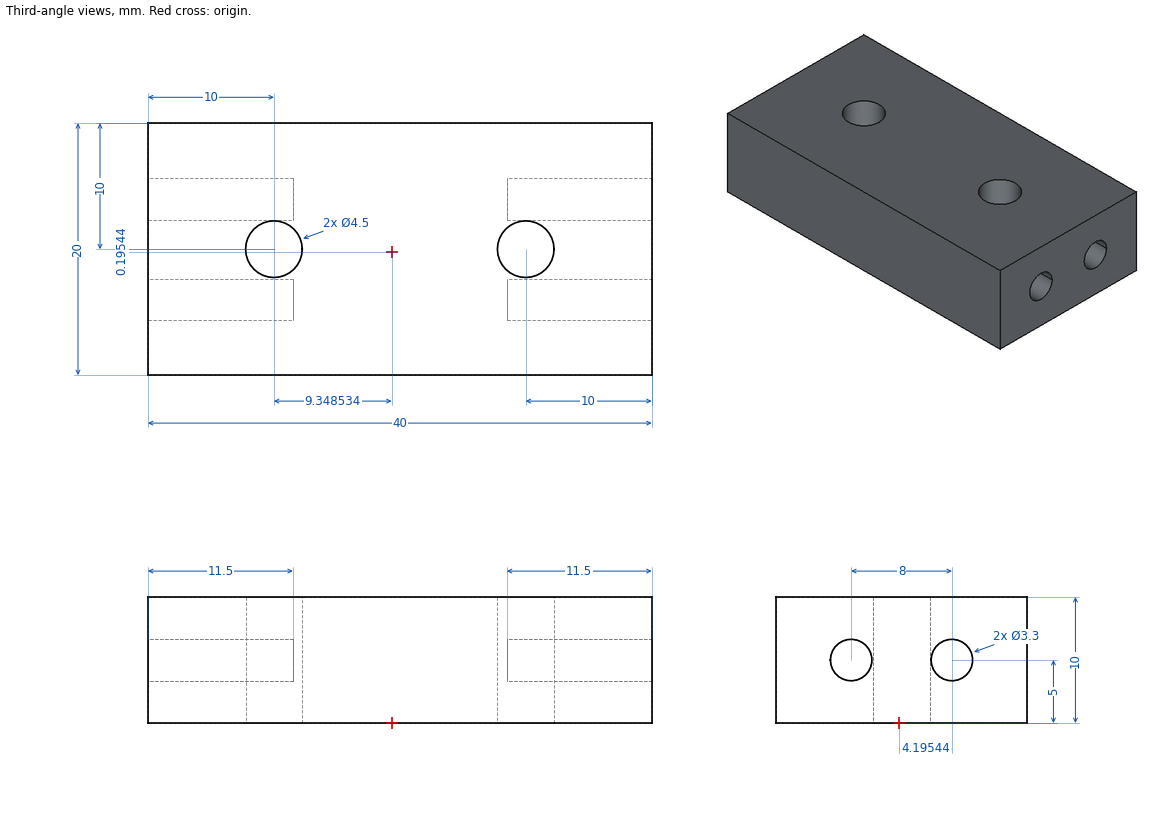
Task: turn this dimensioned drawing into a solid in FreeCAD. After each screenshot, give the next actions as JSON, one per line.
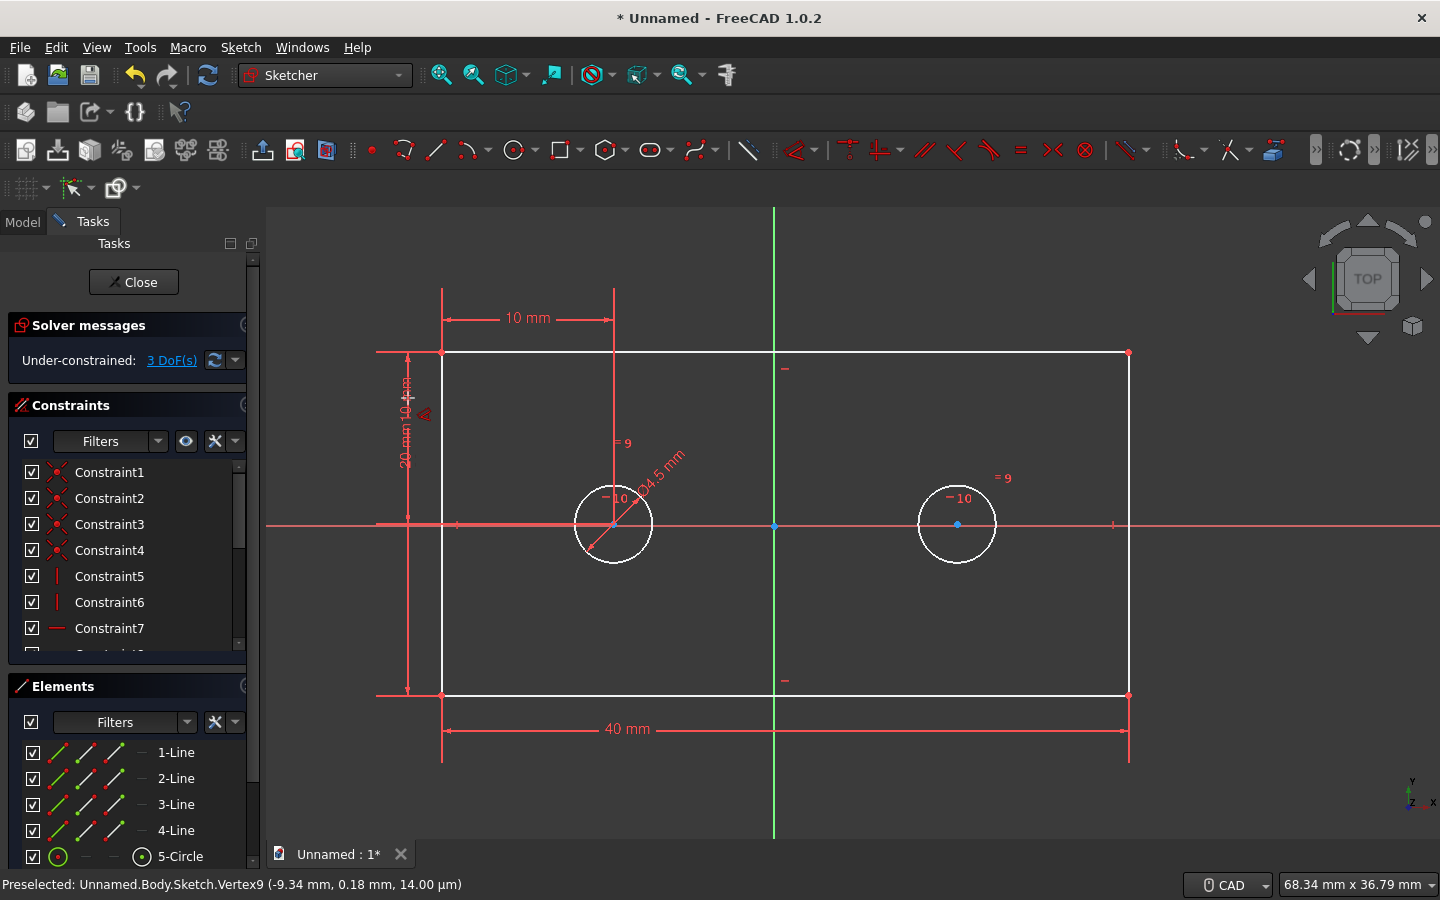
{"action": "left_click", "coordinate": [1129, 696]}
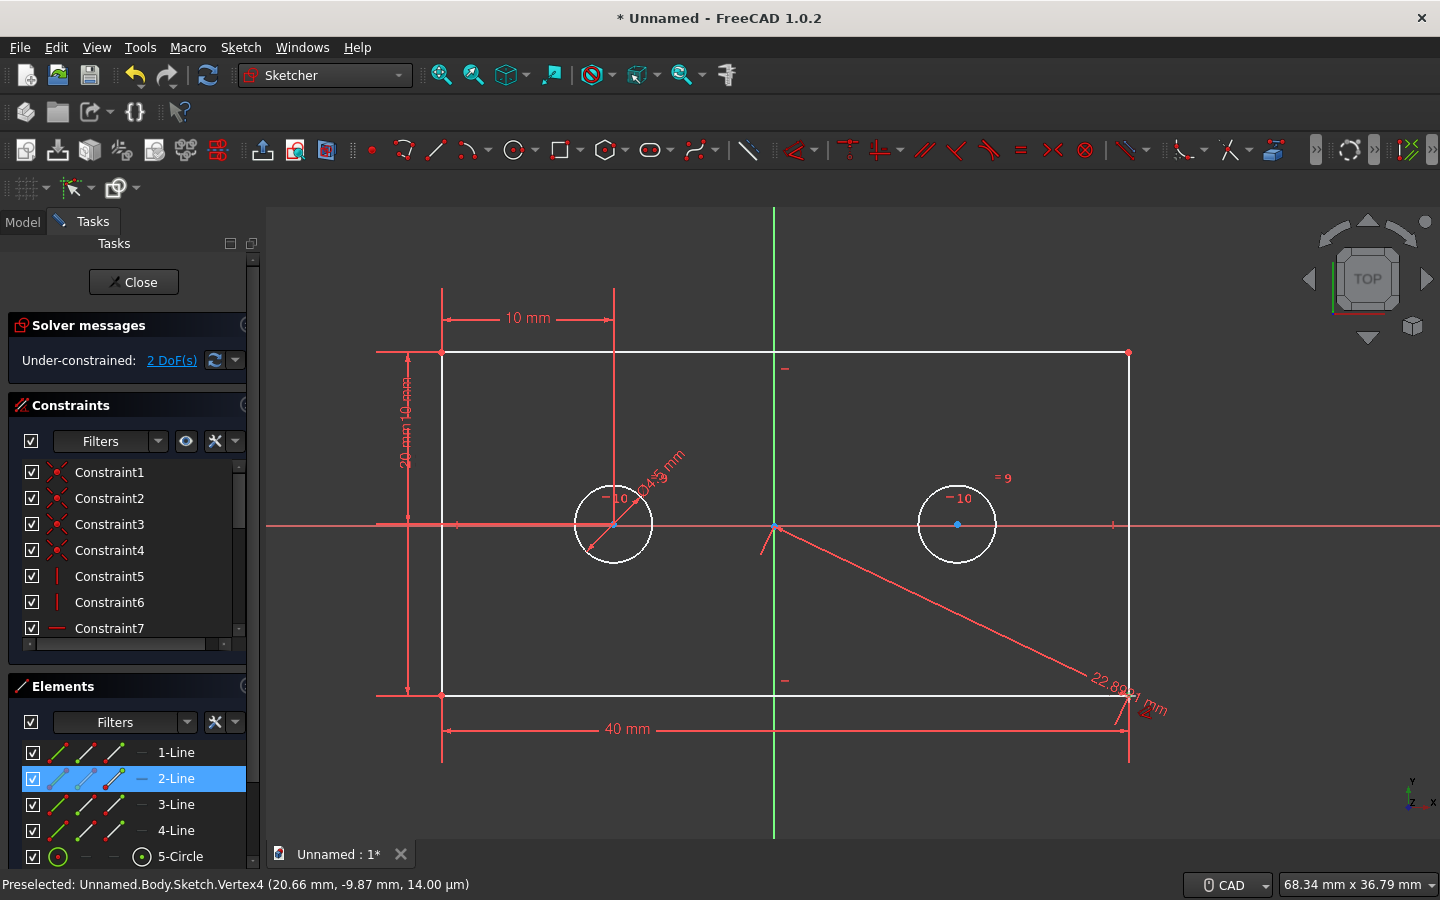
{"action": "left_click", "coordinate": [957, 524]}
{"action": "left_click", "coordinate": [1043, 730]}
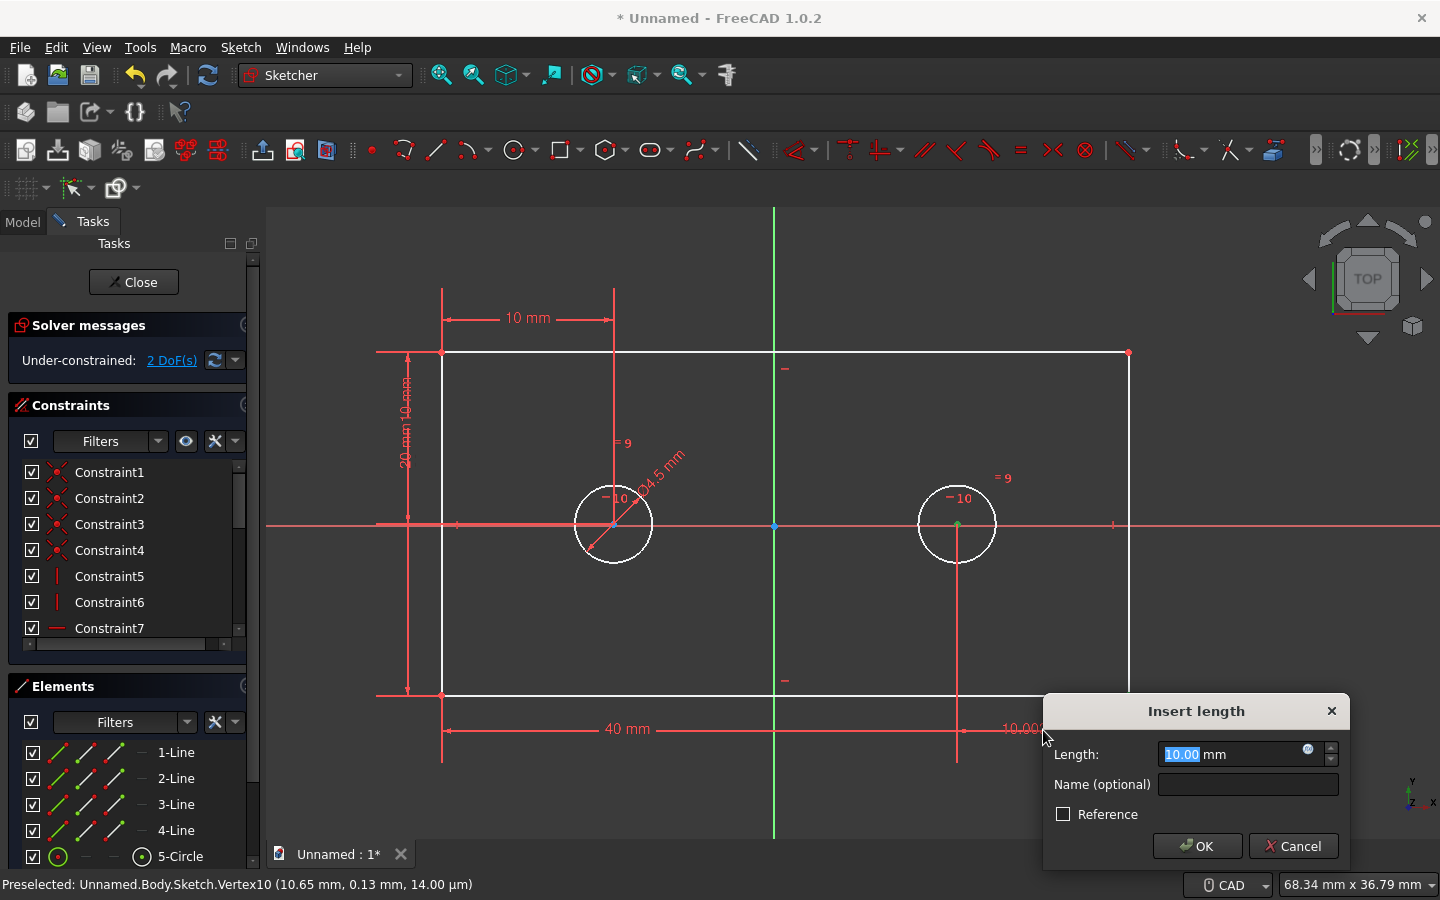
{"action": "type", "text": "10"}
{"action": "key", "text": "Return"}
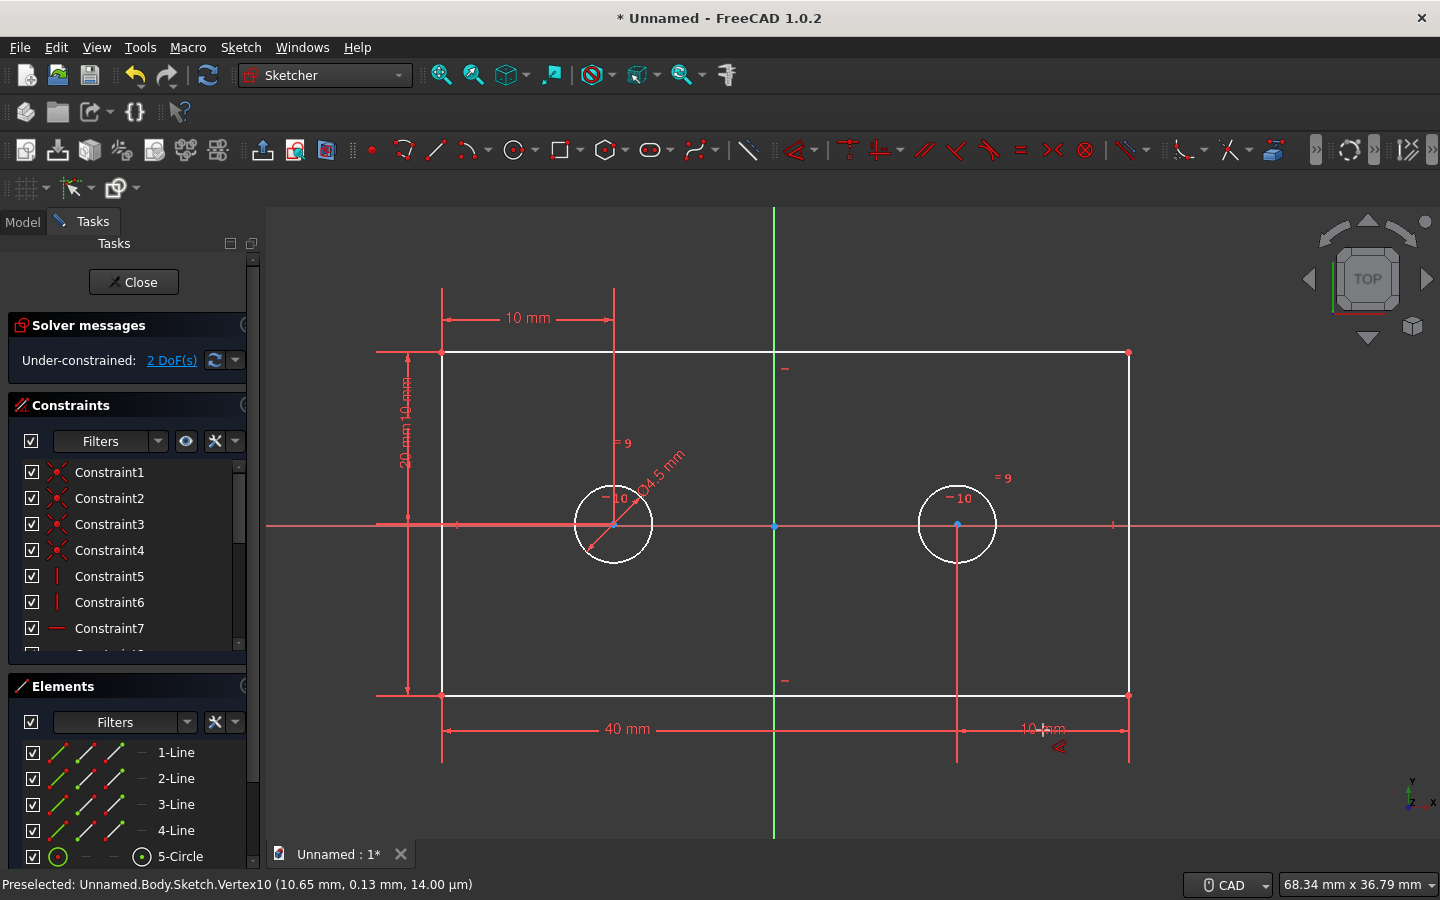
{"action": "scroll", "coordinate": [614, 524], "scroll_direction": "up", "scroll_amount": 13}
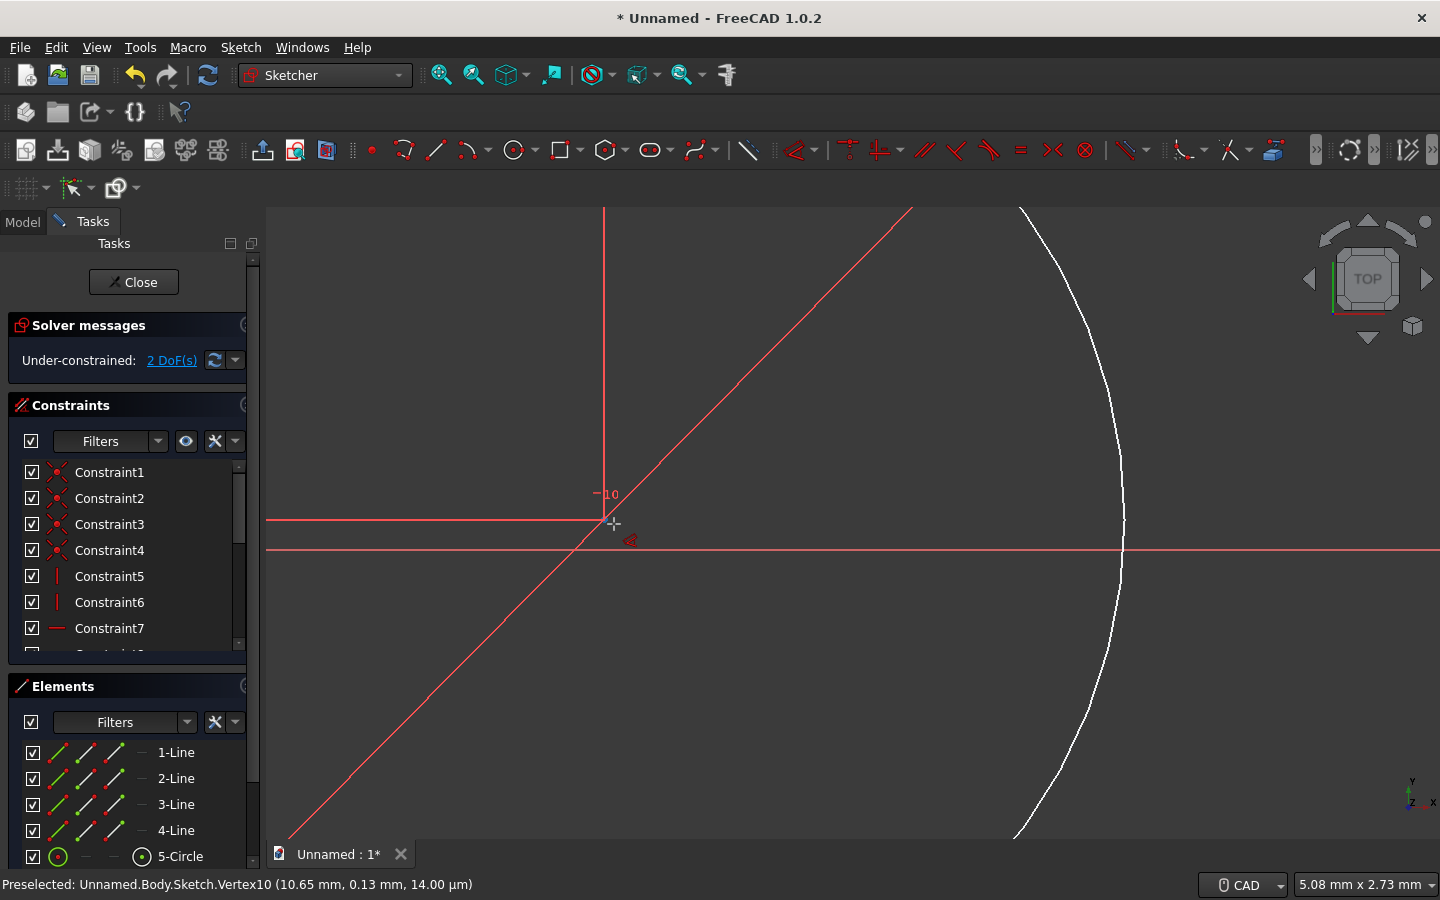
{"action": "left_click", "coordinate": [604, 520]}
{"action": "left_click", "coordinate": [570, 535]}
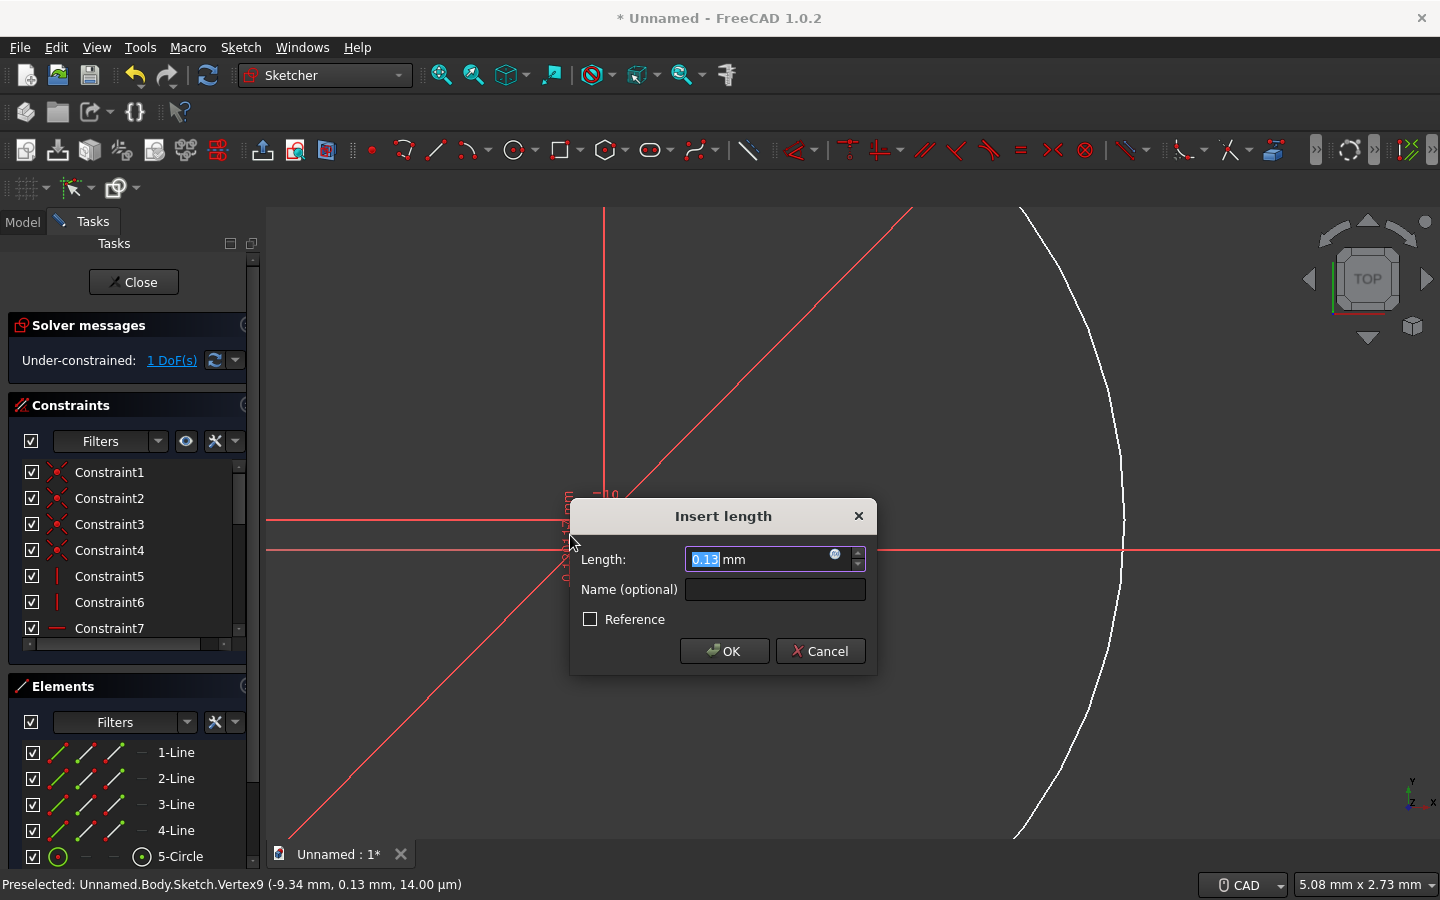
{"action": "type", "text": "0.19544"}
{"action": "key", "text": "Return"}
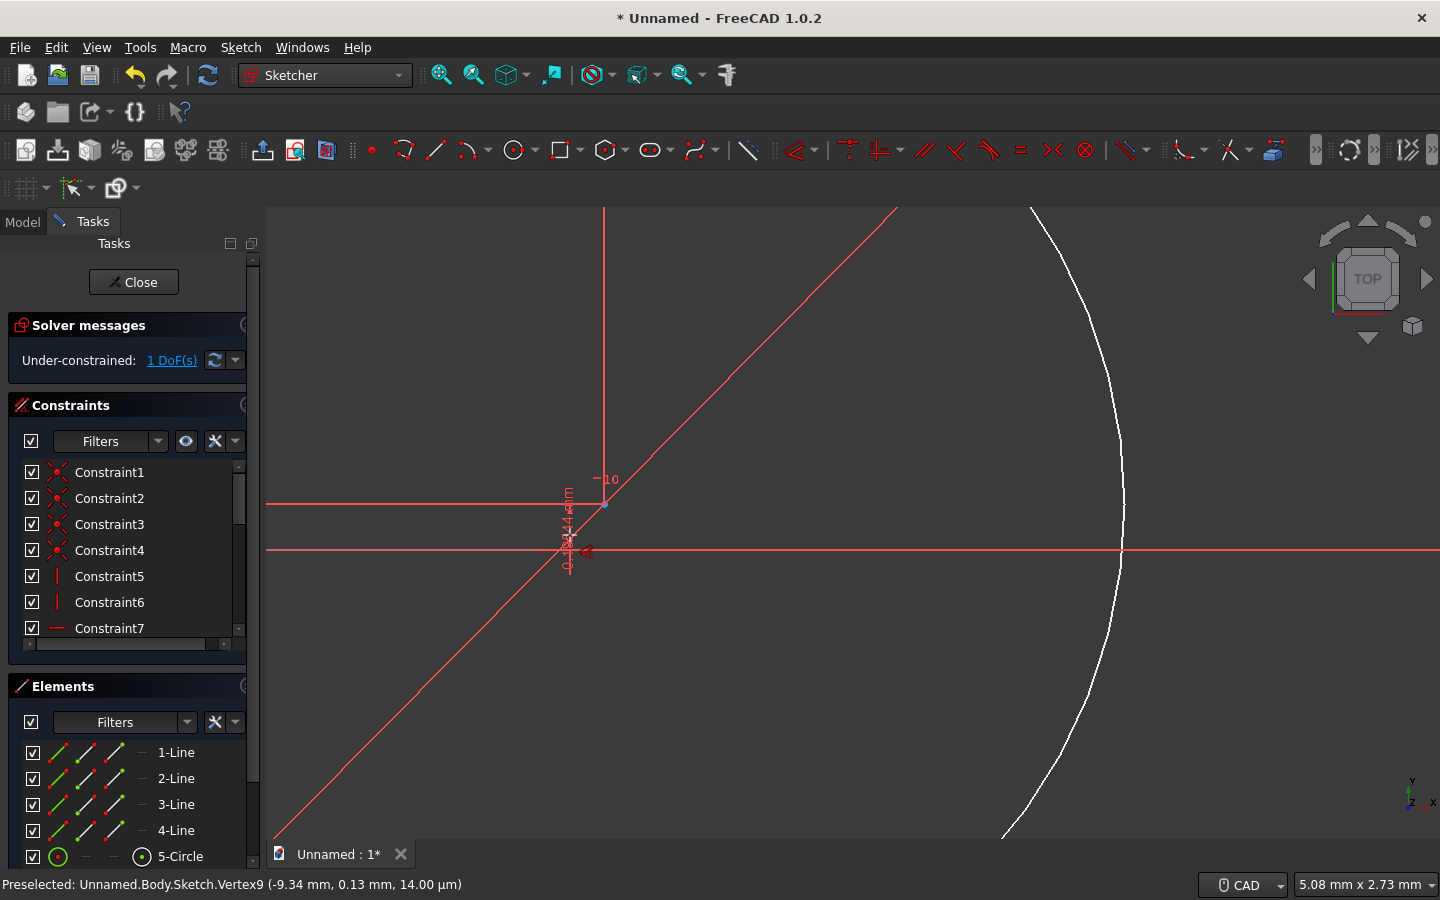
{"action": "scroll", "coordinate": [613, 524], "scroll_direction": "down", "scroll_amount": 13}